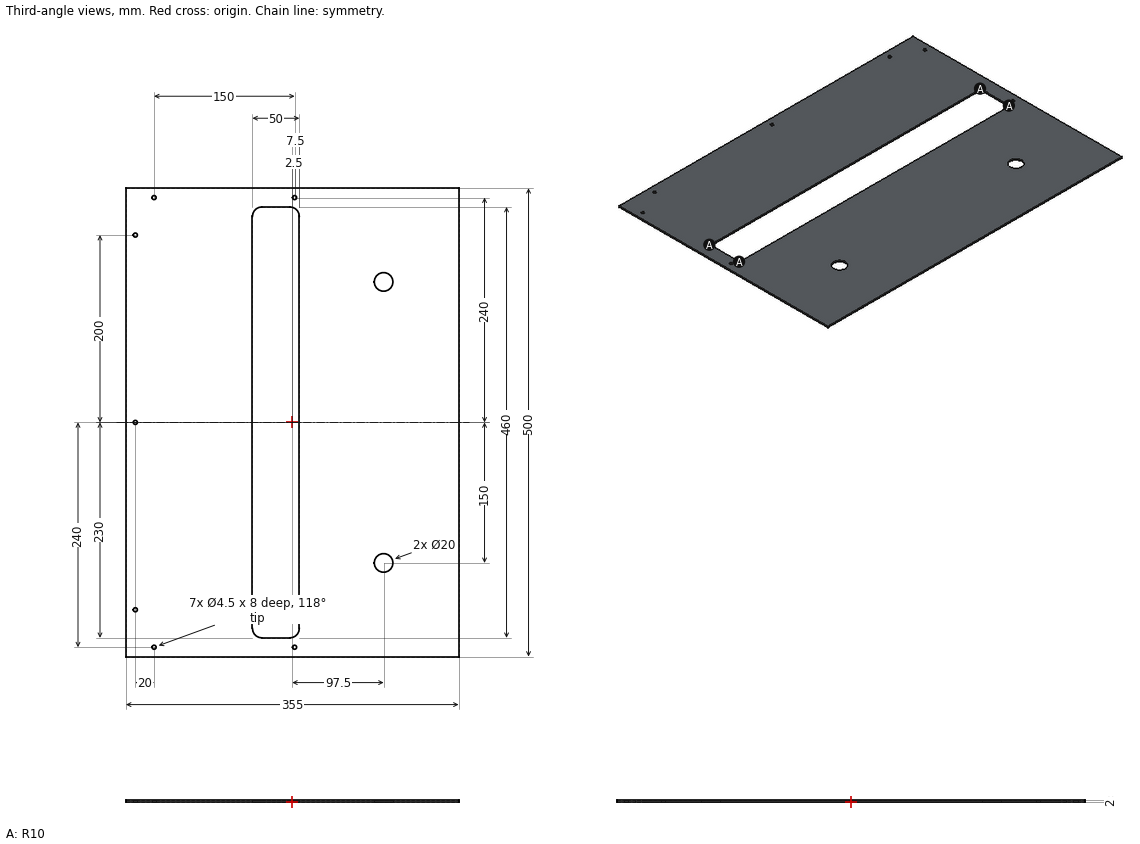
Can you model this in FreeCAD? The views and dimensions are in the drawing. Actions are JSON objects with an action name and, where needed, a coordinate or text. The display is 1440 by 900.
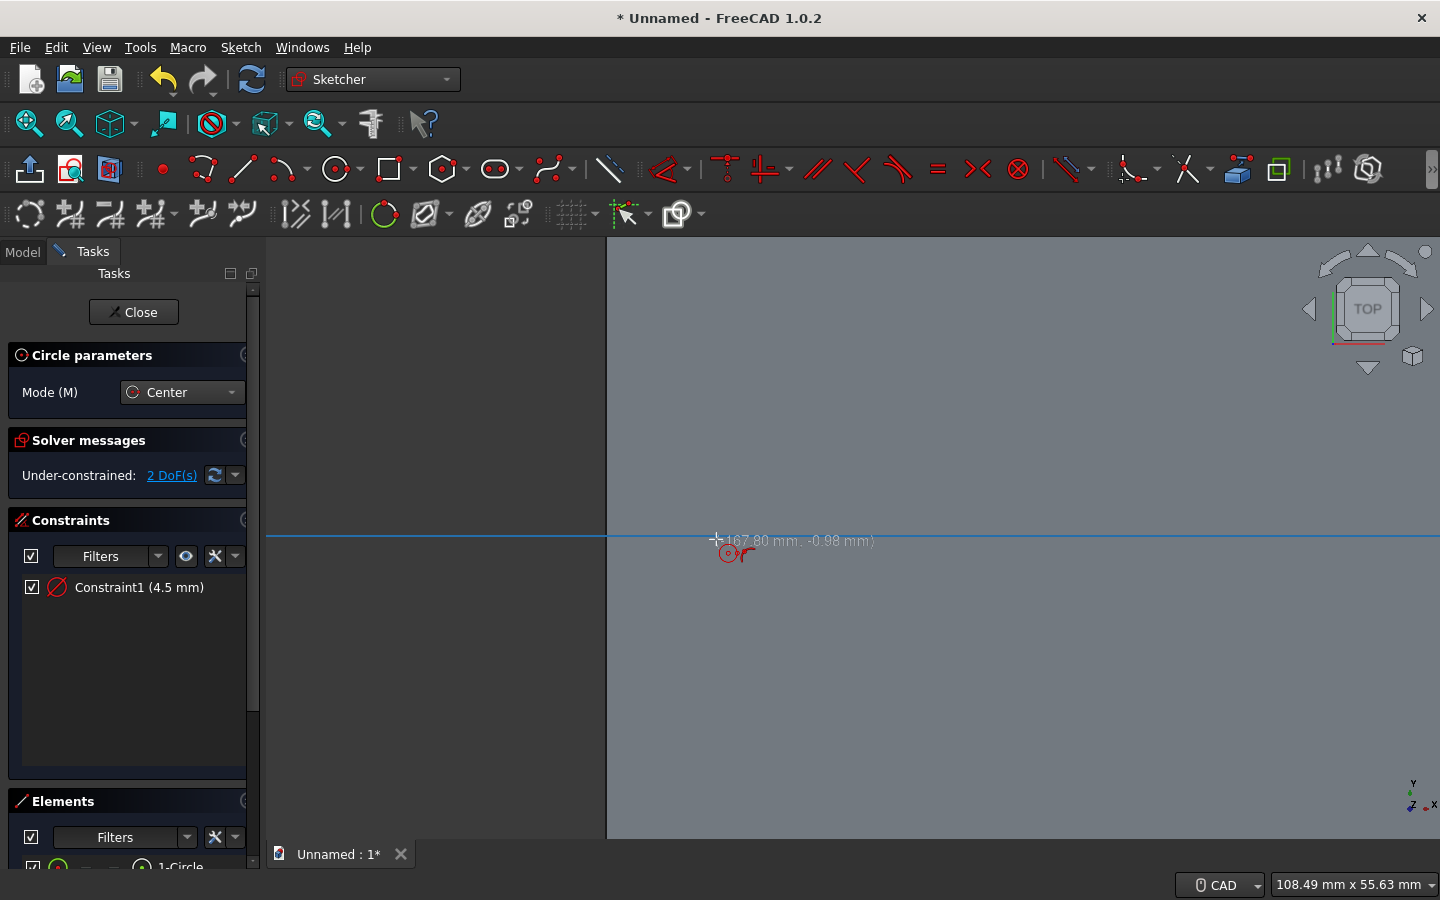
{"action": "scroll", "coordinate": [716, 538], "scroll_direction": "down", "scroll_amount": 13}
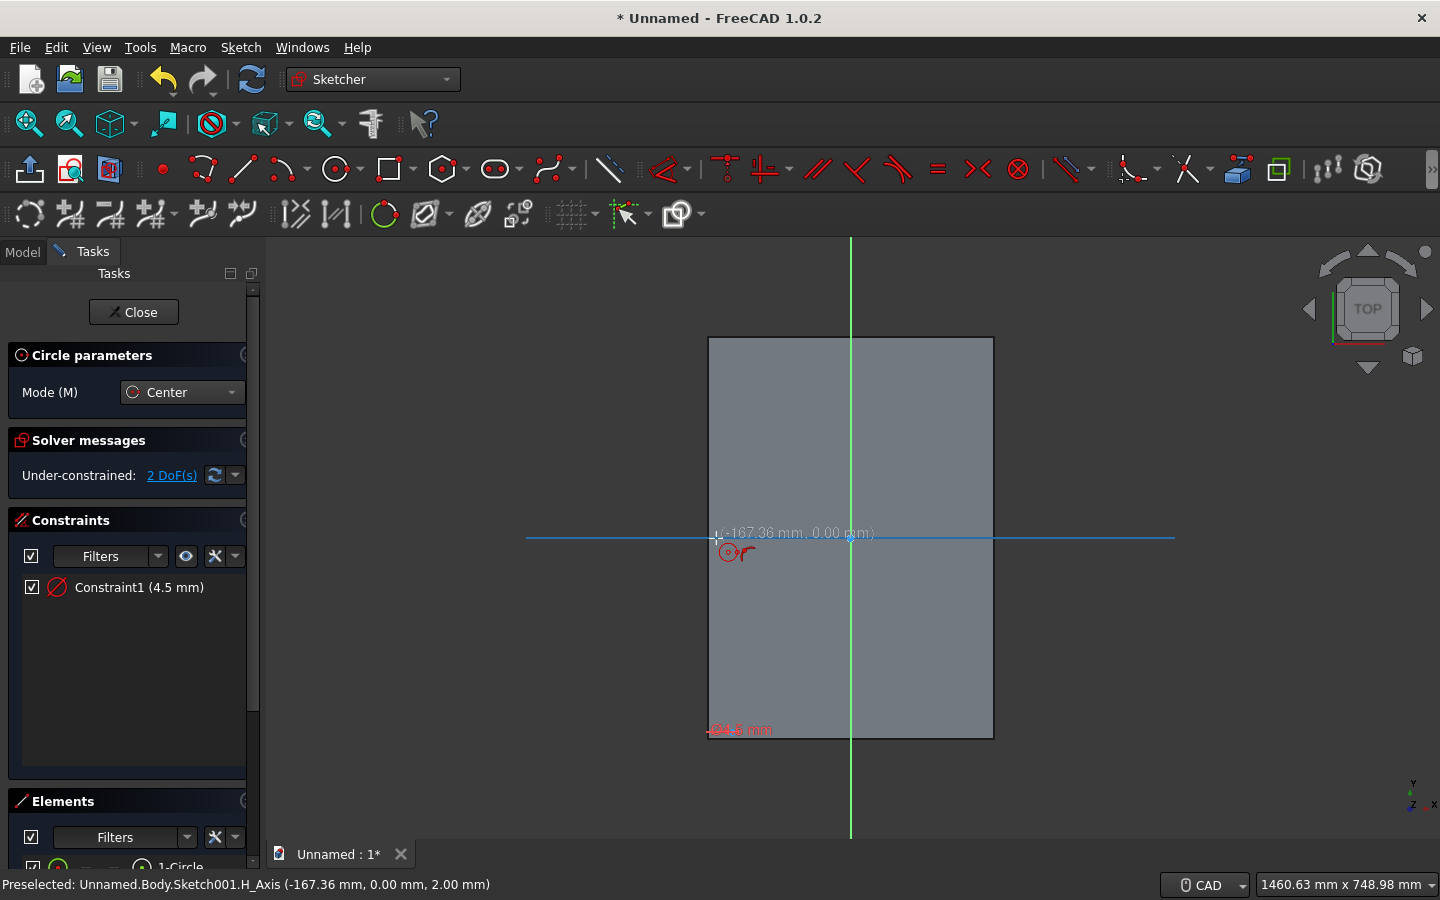
{"action": "left_click", "coordinate": [716, 538]}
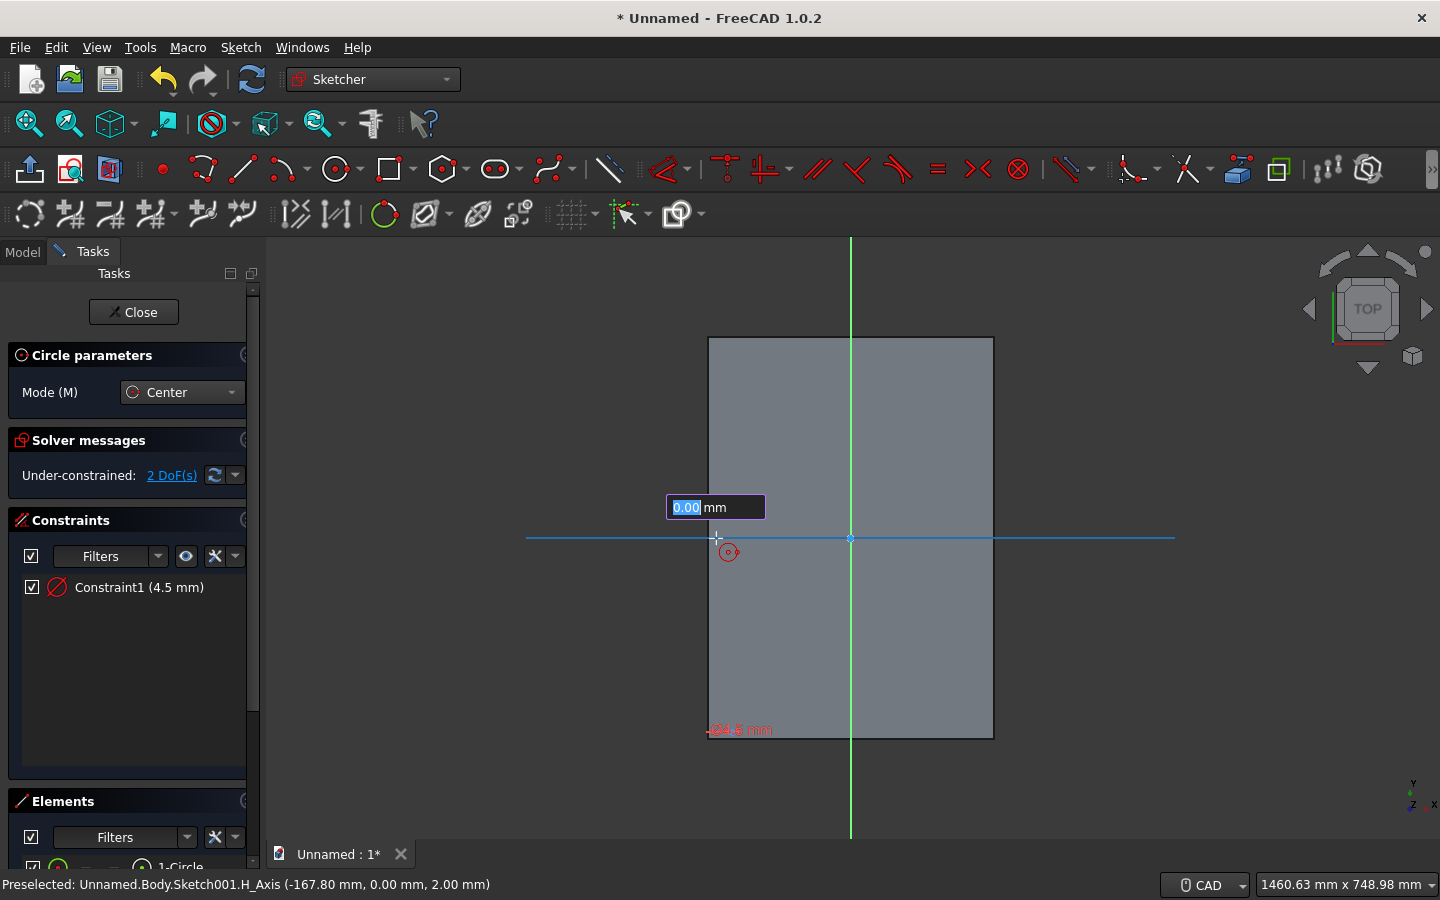
{"action": "scroll", "coordinate": [716, 540], "scroll_direction": "up", "scroll_amount": 12}
{"action": "mouse_move", "coordinate": [708, 535]}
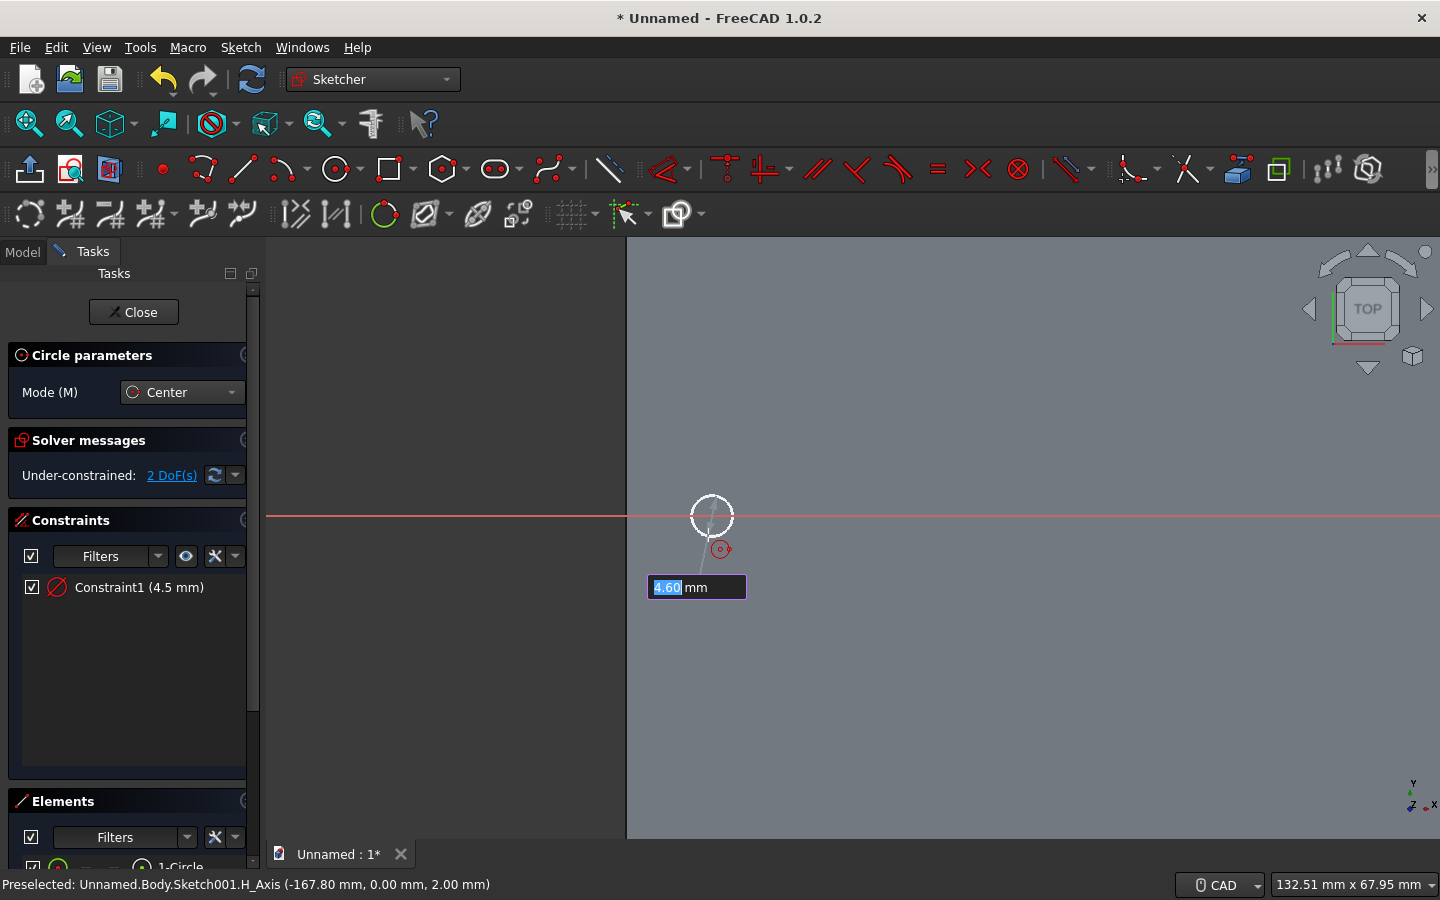
{"action": "type", "text": "4.5"}
{"action": "key", "text": "Return"}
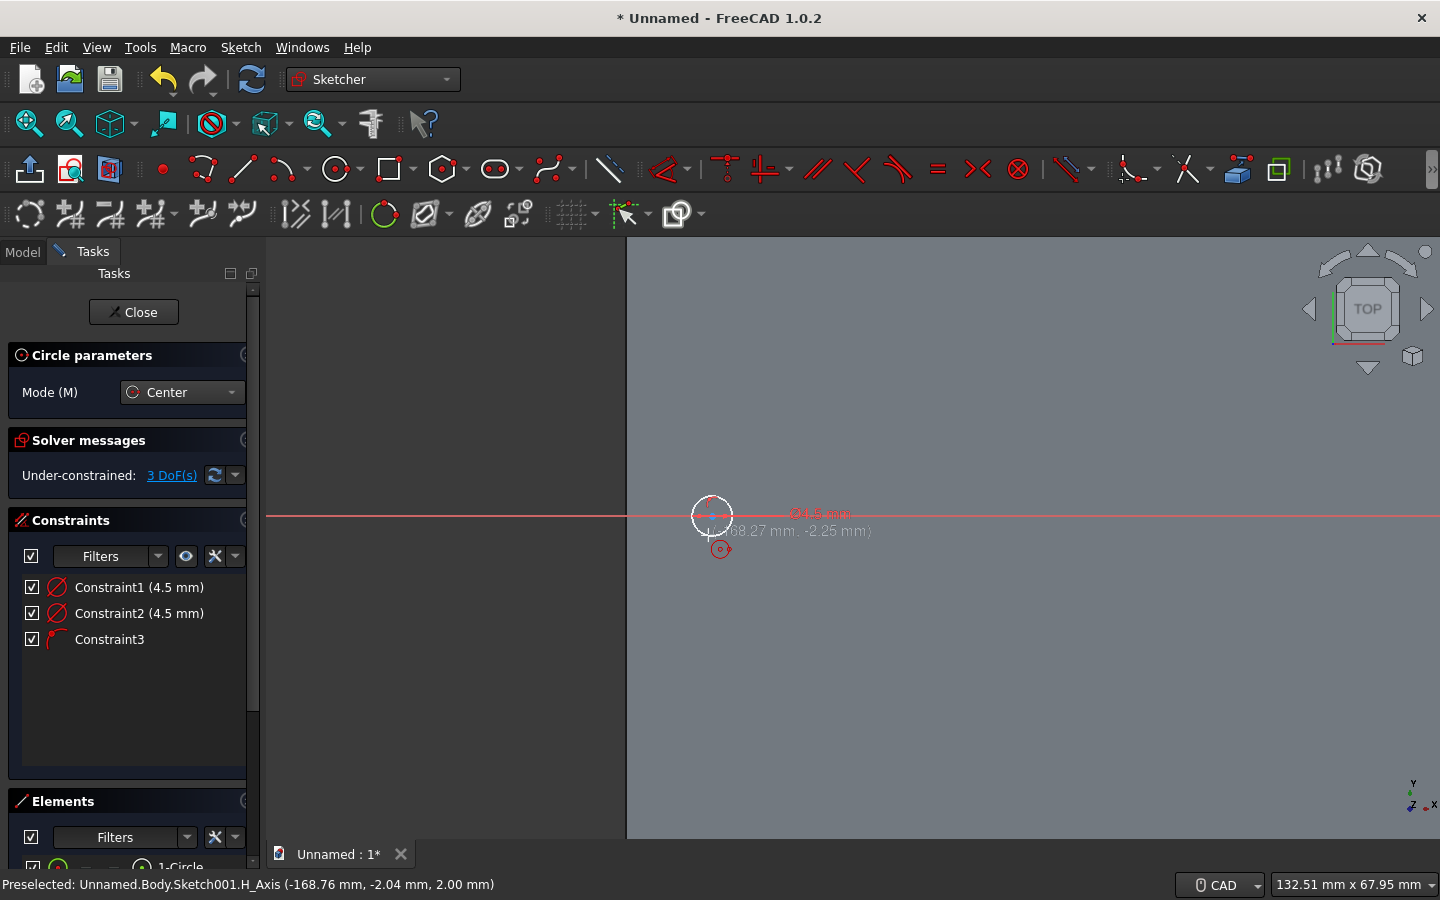
{"action": "scroll", "coordinate": [716, 540], "scroll_direction": "down", "scroll_amount": 12}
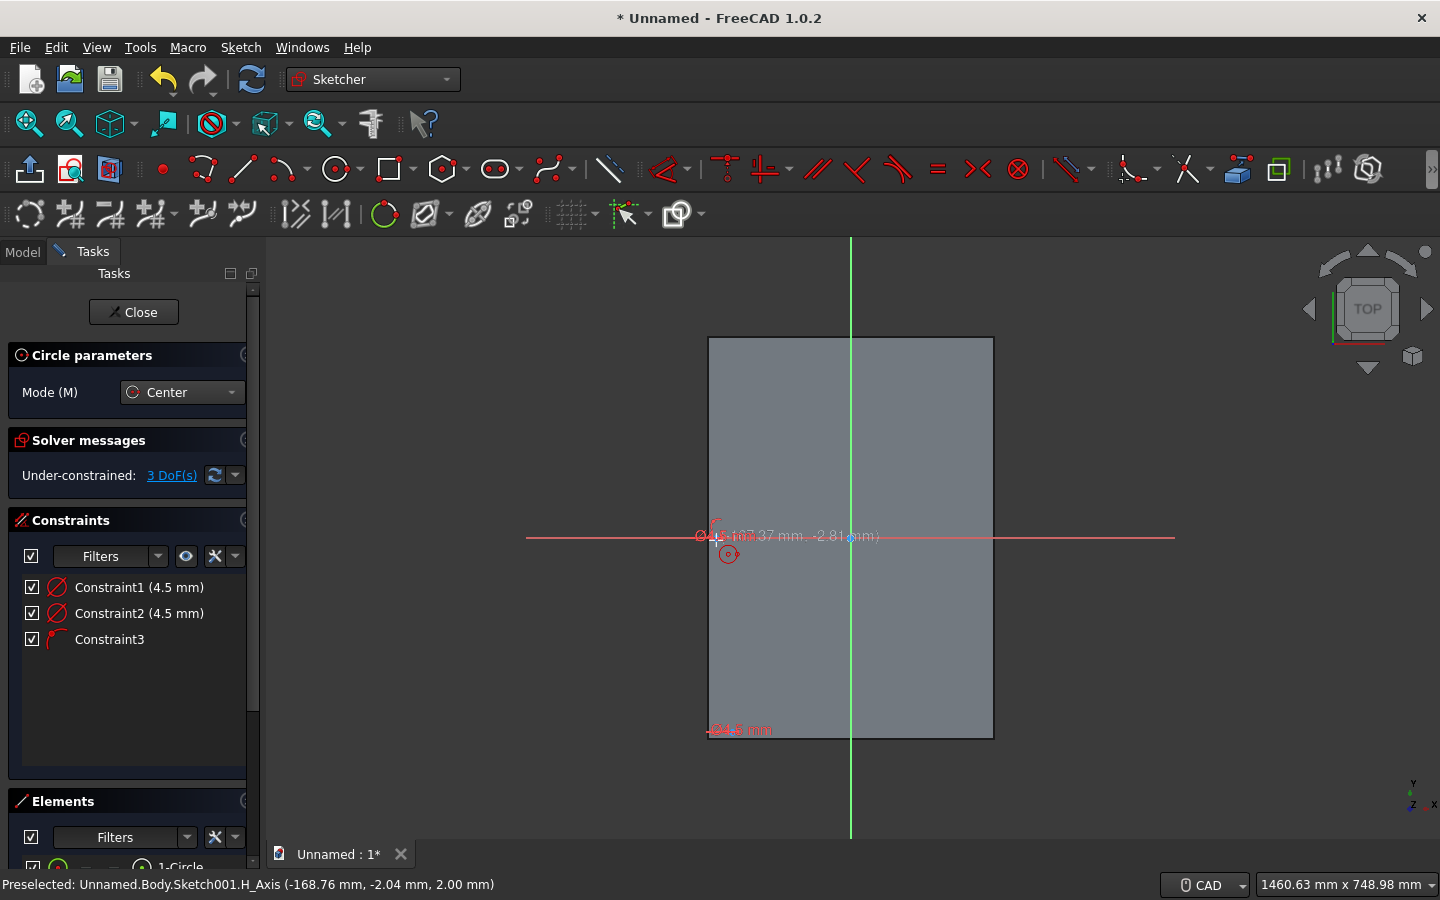
{"action": "scroll", "coordinate": [716, 378], "scroll_direction": "up", "scroll_amount": 13}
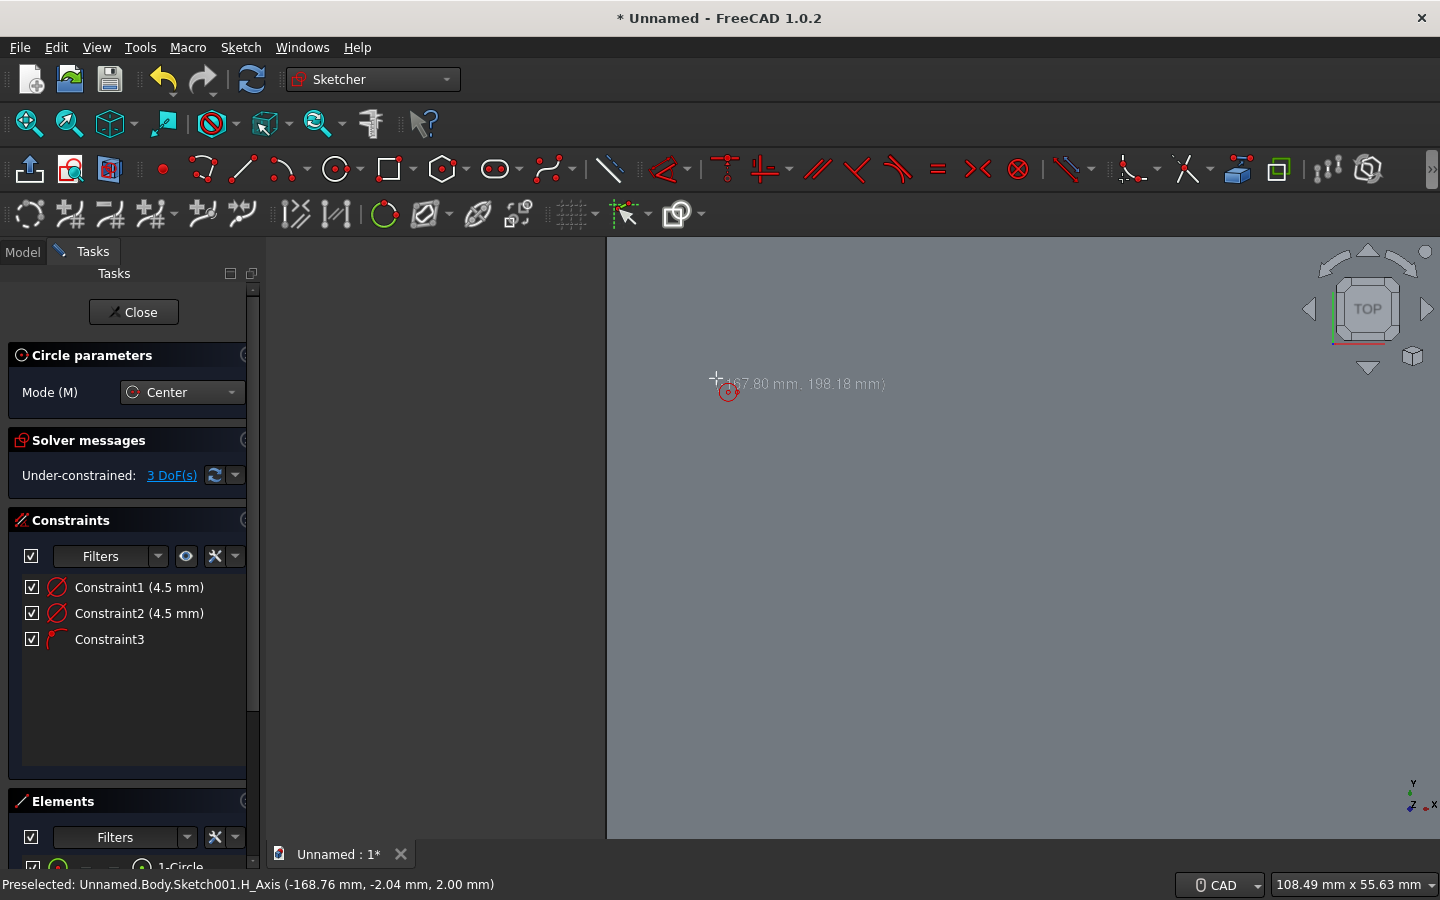
{"action": "scroll", "coordinate": [716, 378], "scroll_direction": "down", "scroll_amount": 13}